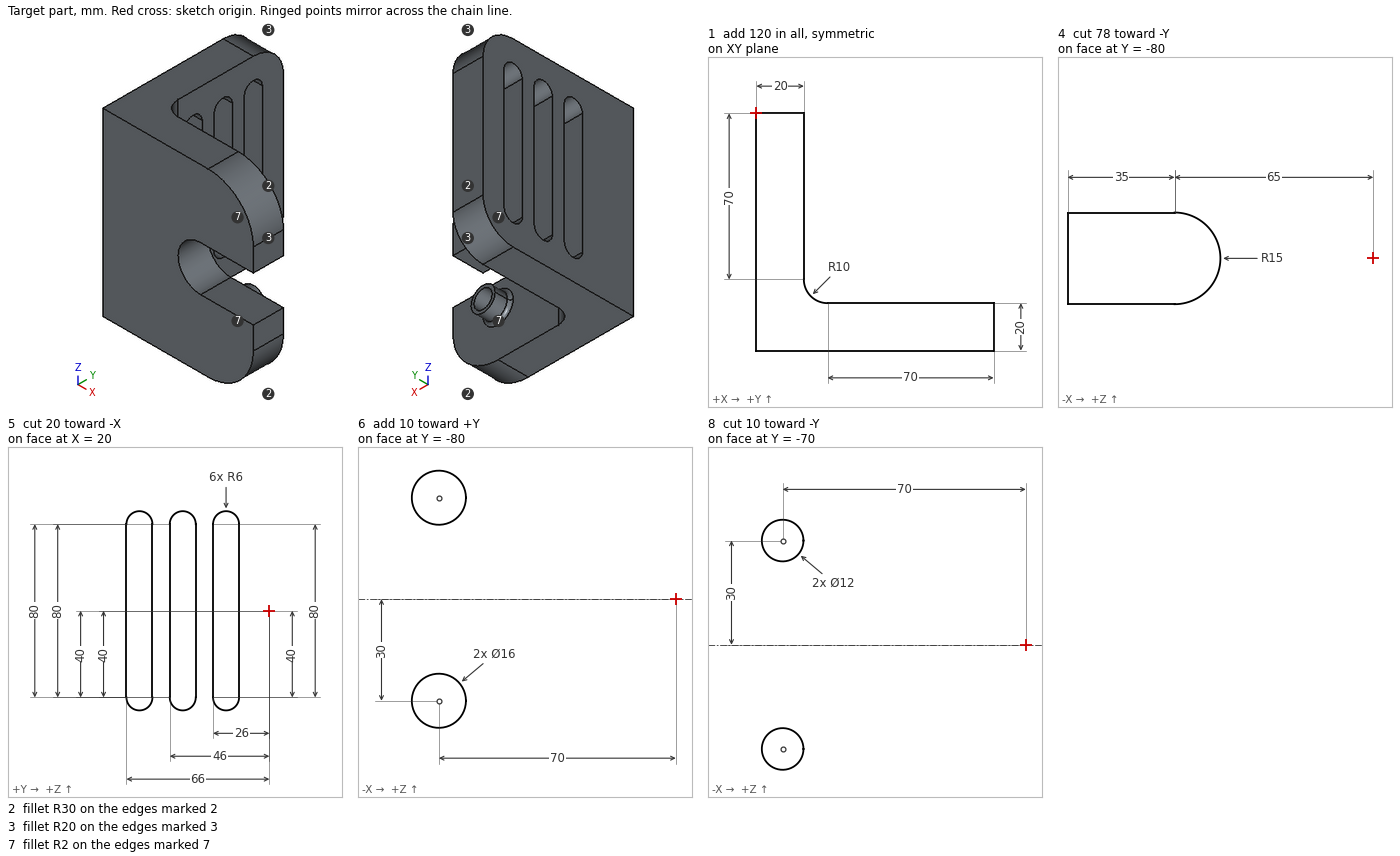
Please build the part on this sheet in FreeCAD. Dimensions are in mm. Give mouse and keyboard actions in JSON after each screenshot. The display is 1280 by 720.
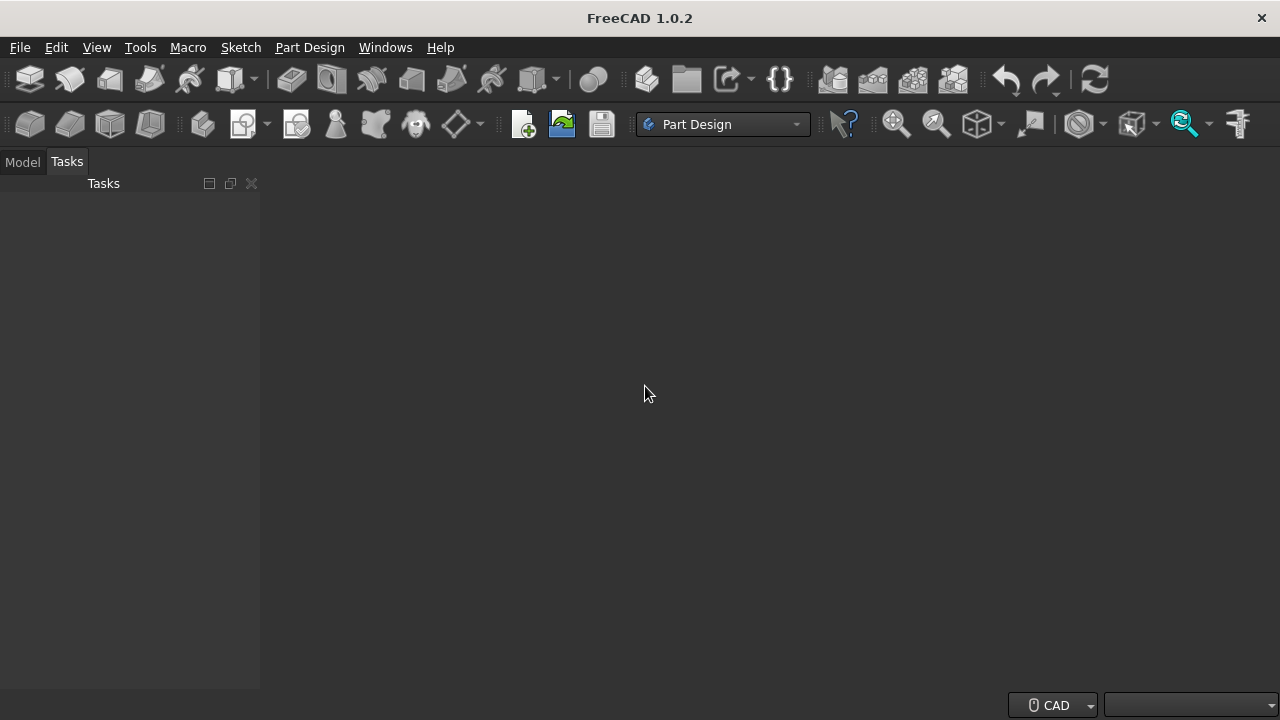
{"action": "key", "text": "ctrl+n"}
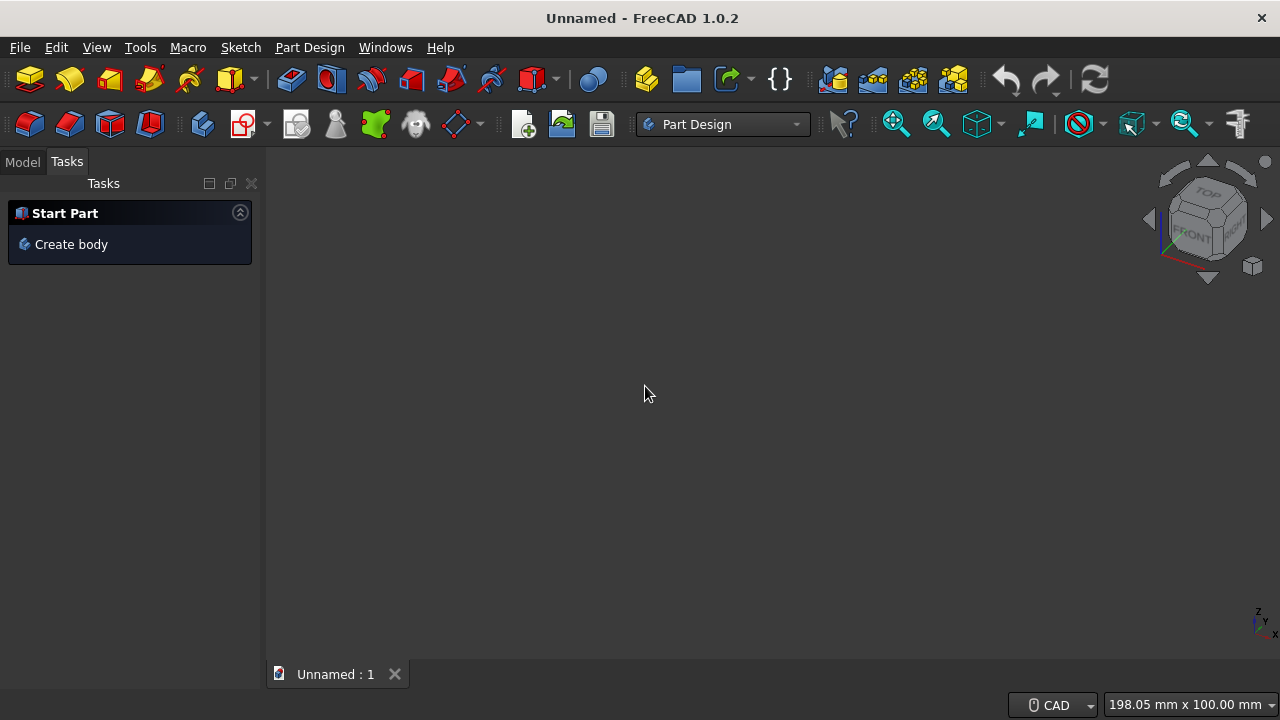
{"action": "left_click", "coordinate": [244, 124]}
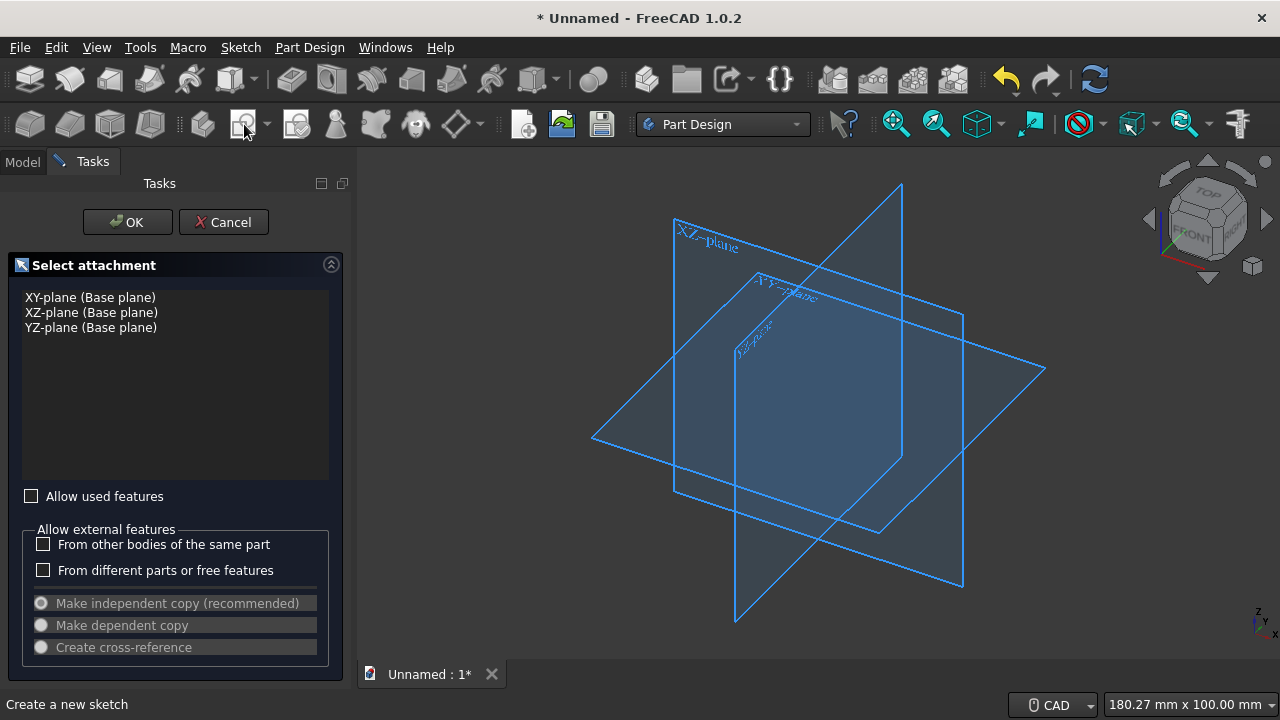
{"action": "left_click", "coordinate": [82, 298]}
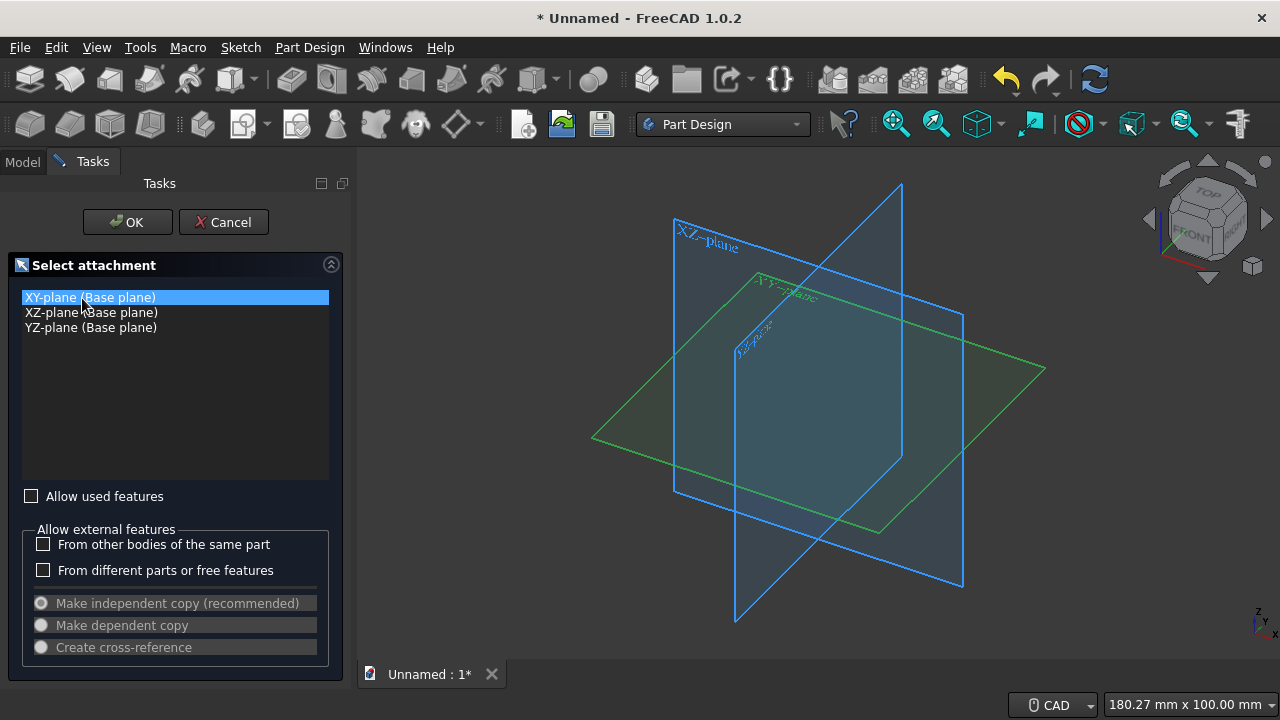
{"action": "left_click", "coordinate": [128, 222]}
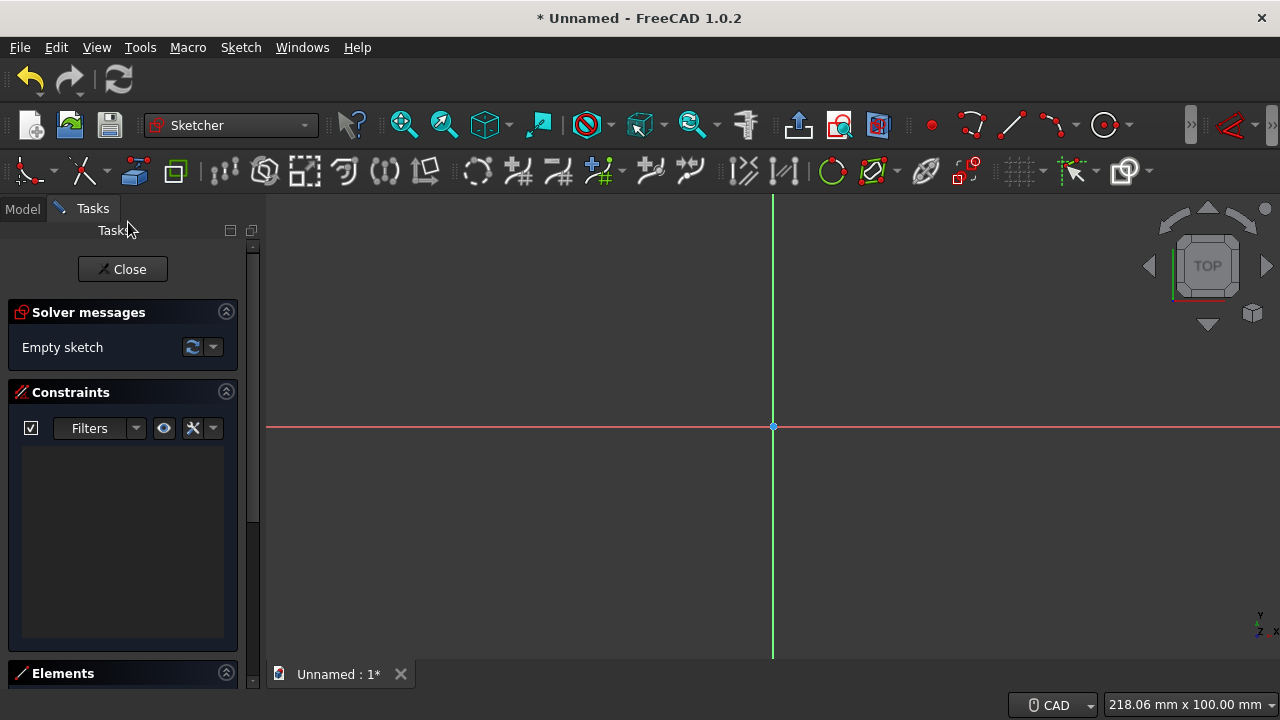
{"action": "scroll", "coordinate": [338, 222], "scroll_direction": "down", "scroll_amount": 3}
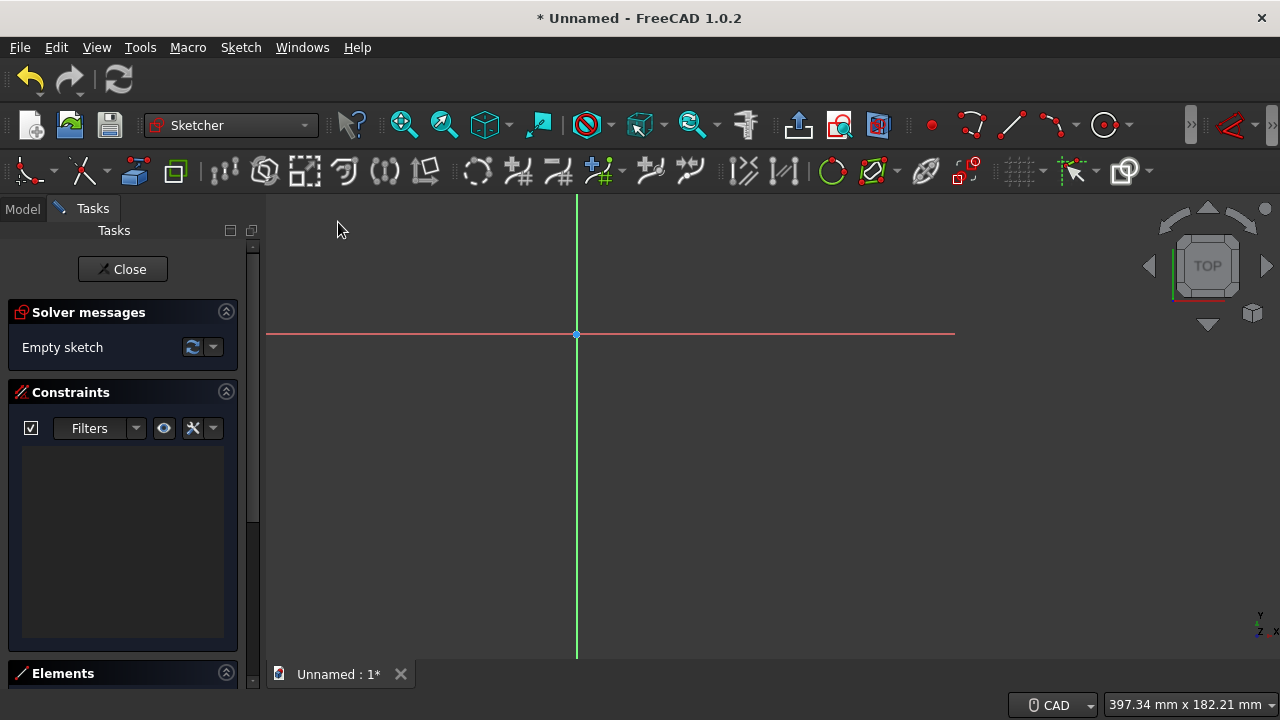
{"action": "left_click", "coordinate": [972, 126]}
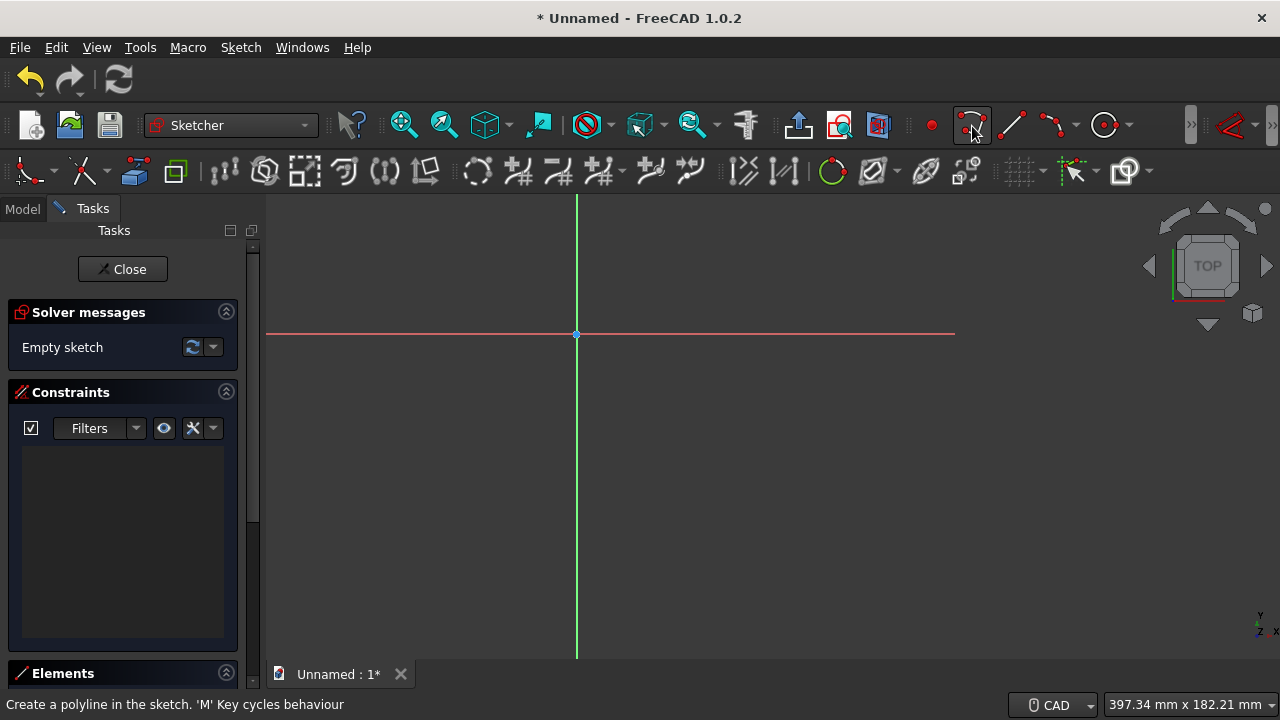
{"action": "left_click", "coordinate": [628, 513]}
{"action": "left_click", "coordinate": [628, 334]}
{"action": "left_click", "coordinate": [577, 334]}
{"action": "left_click", "coordinate": [586, 589]}
{"action": "left_click", "coordinate": [832, 589]}
{"action": "left_click", "coordinate": [832, 538]}
{"action": "left_click", "coordinate": [653, 538]}
{"action": "right_click", "coordinate": [653, 538]}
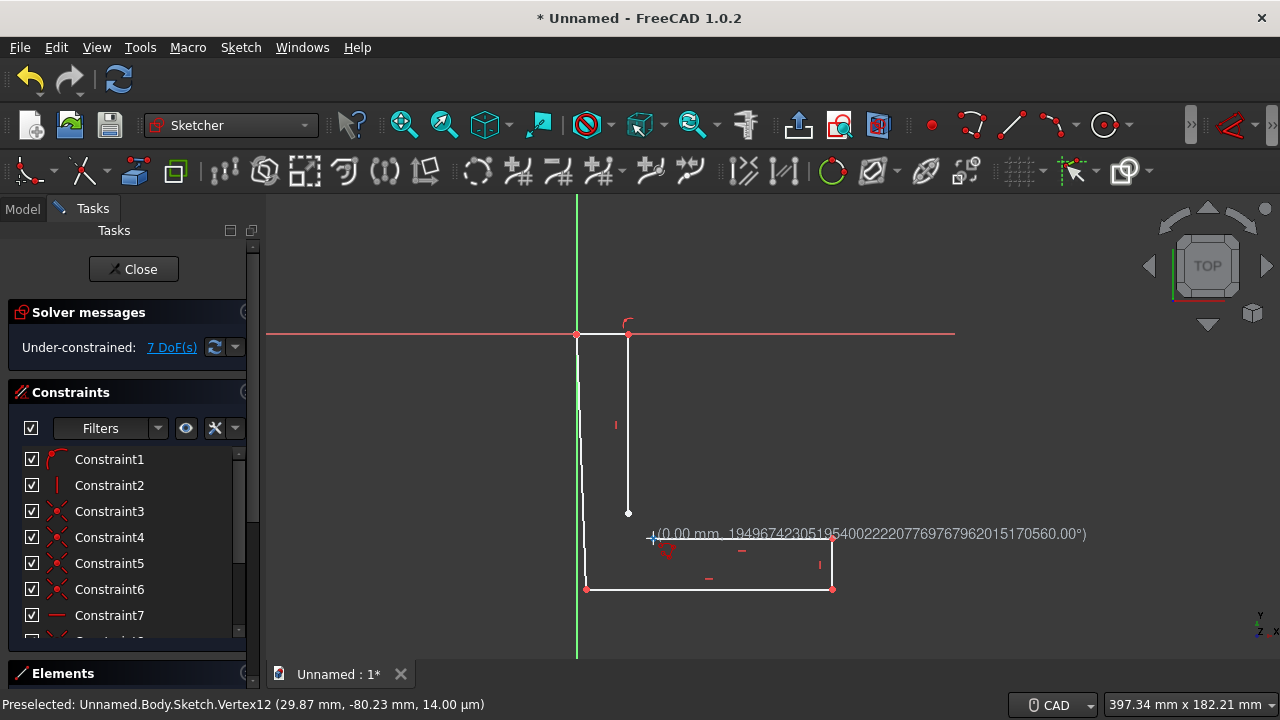
{"action": "left_click", "coordinate": [1052, 126]}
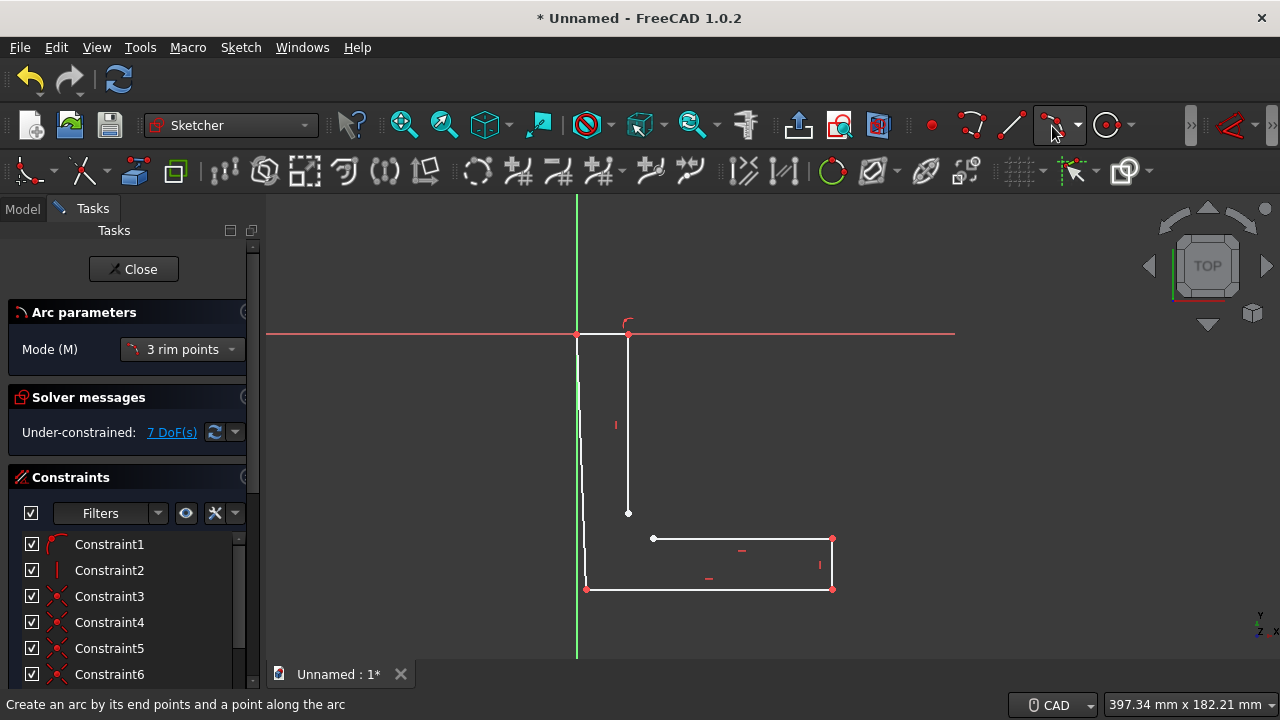
{"action": "left_click", "coordinate": [653, 539]}
{"action": "left_click", "coordinate": [628, 514]}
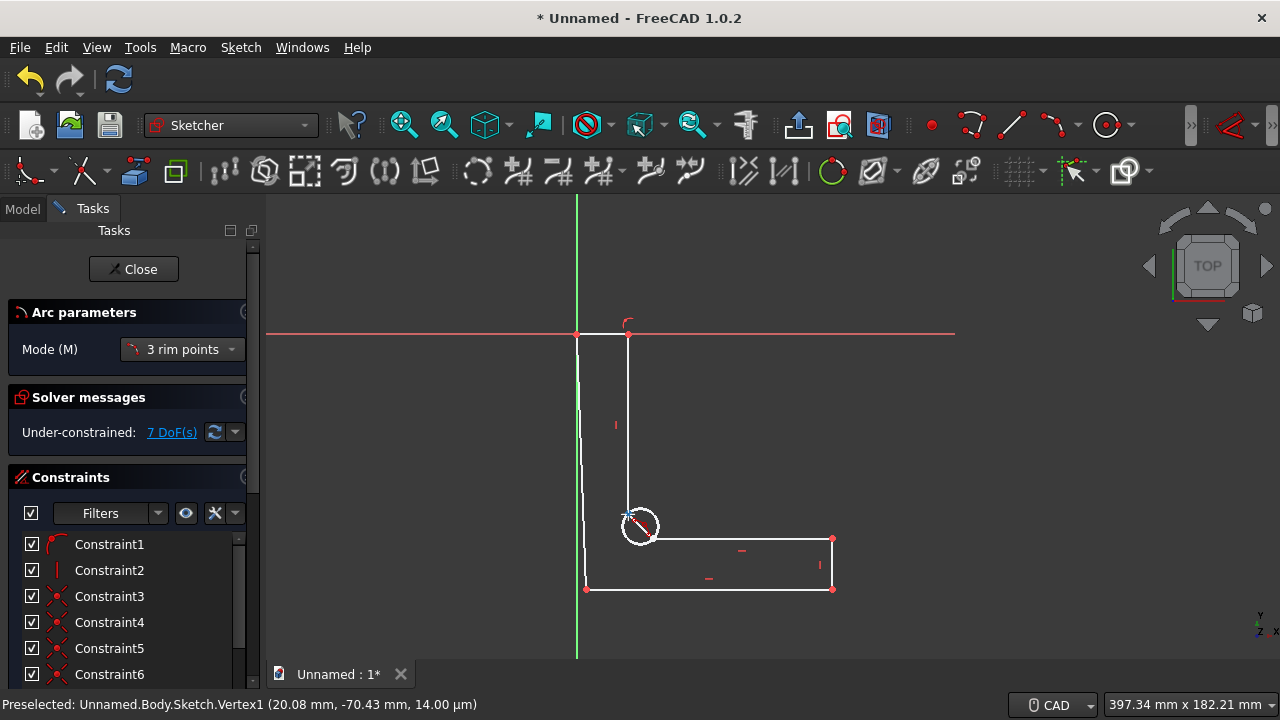
{"action": "scroll", "coordinate": [635, 531], "scroll_direction": "up", "scroll_amount": 4}